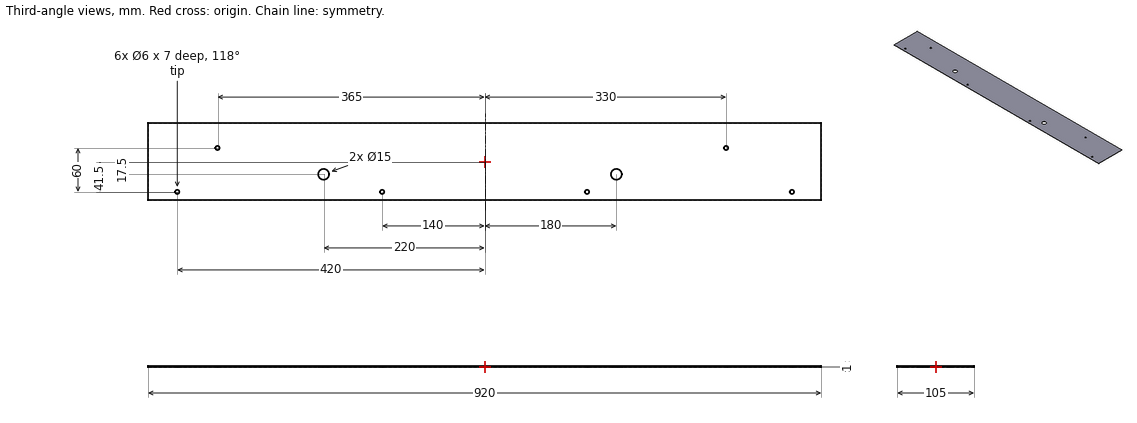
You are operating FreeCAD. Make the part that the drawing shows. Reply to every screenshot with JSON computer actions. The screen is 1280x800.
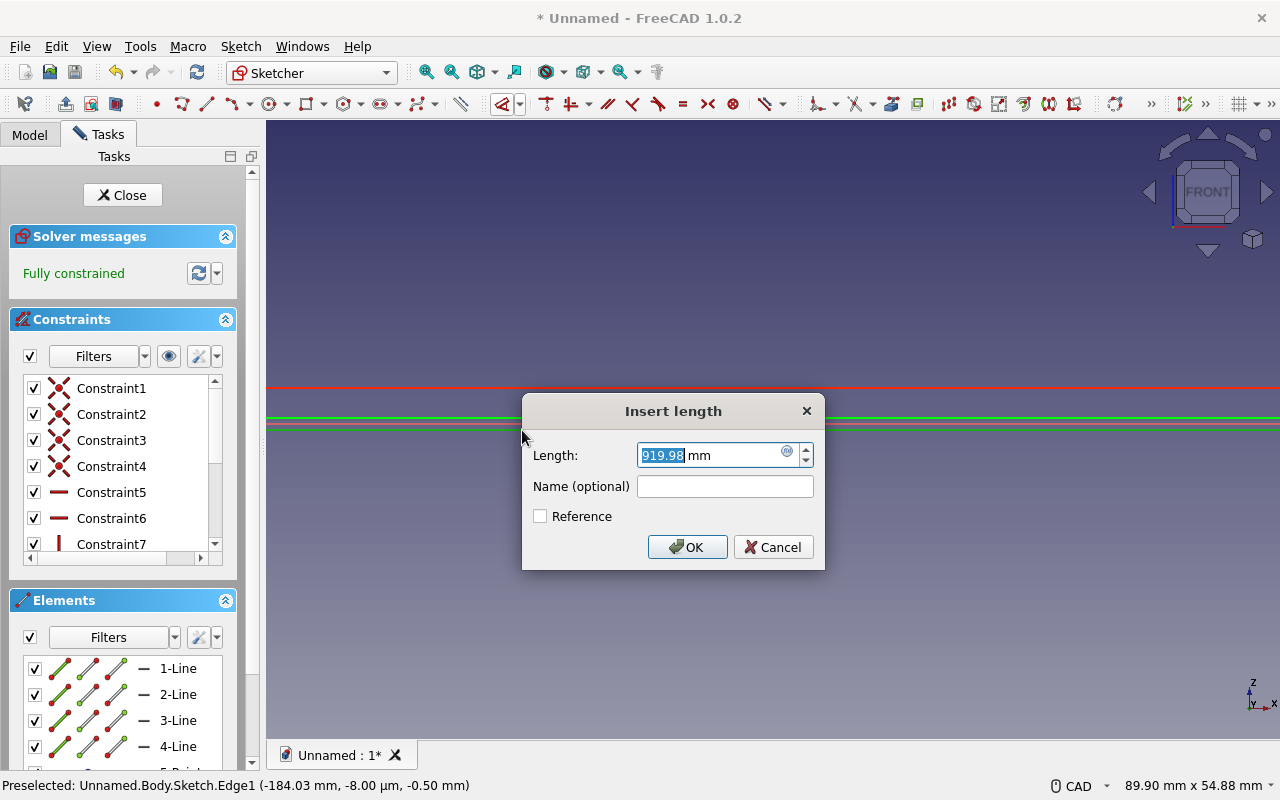
{"action": "type", "text": "920"}
{"action": "key", "text": "Return"}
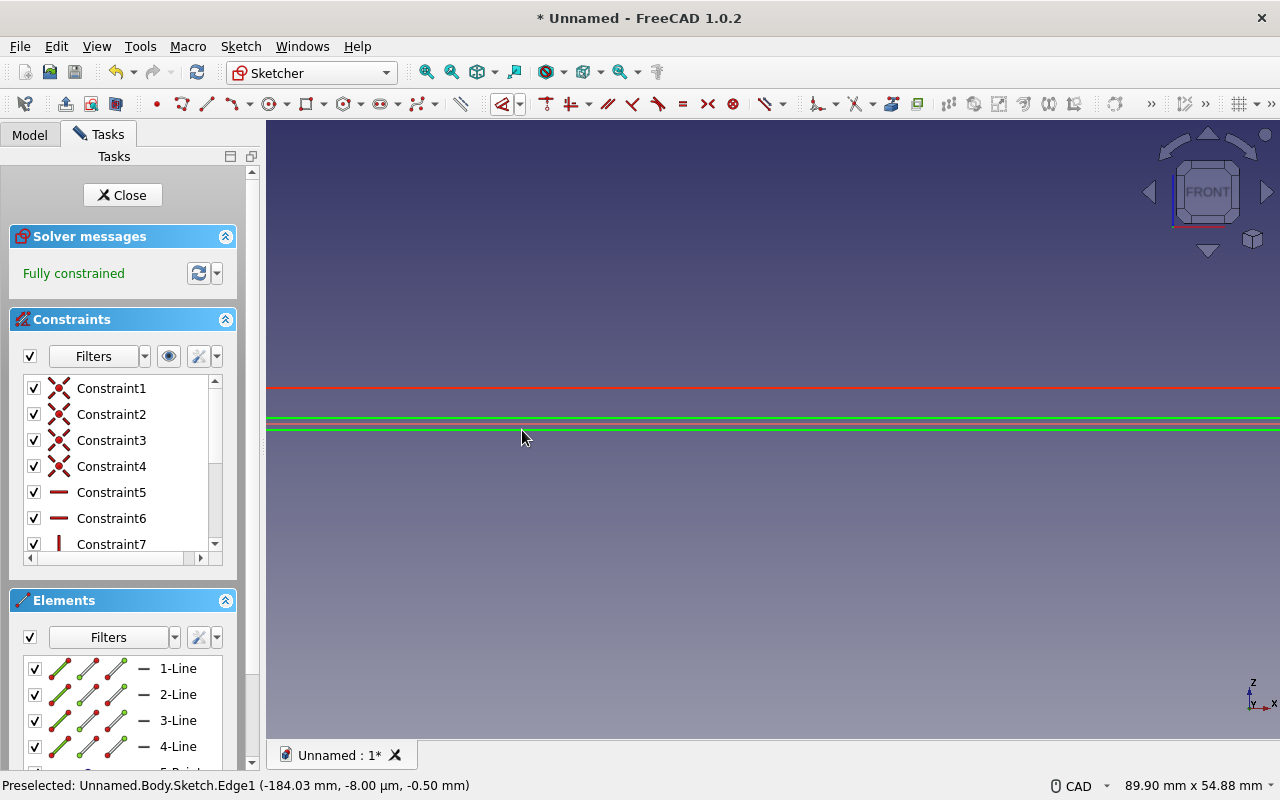
{"action": "left_click", "coordinate": [123, 195]}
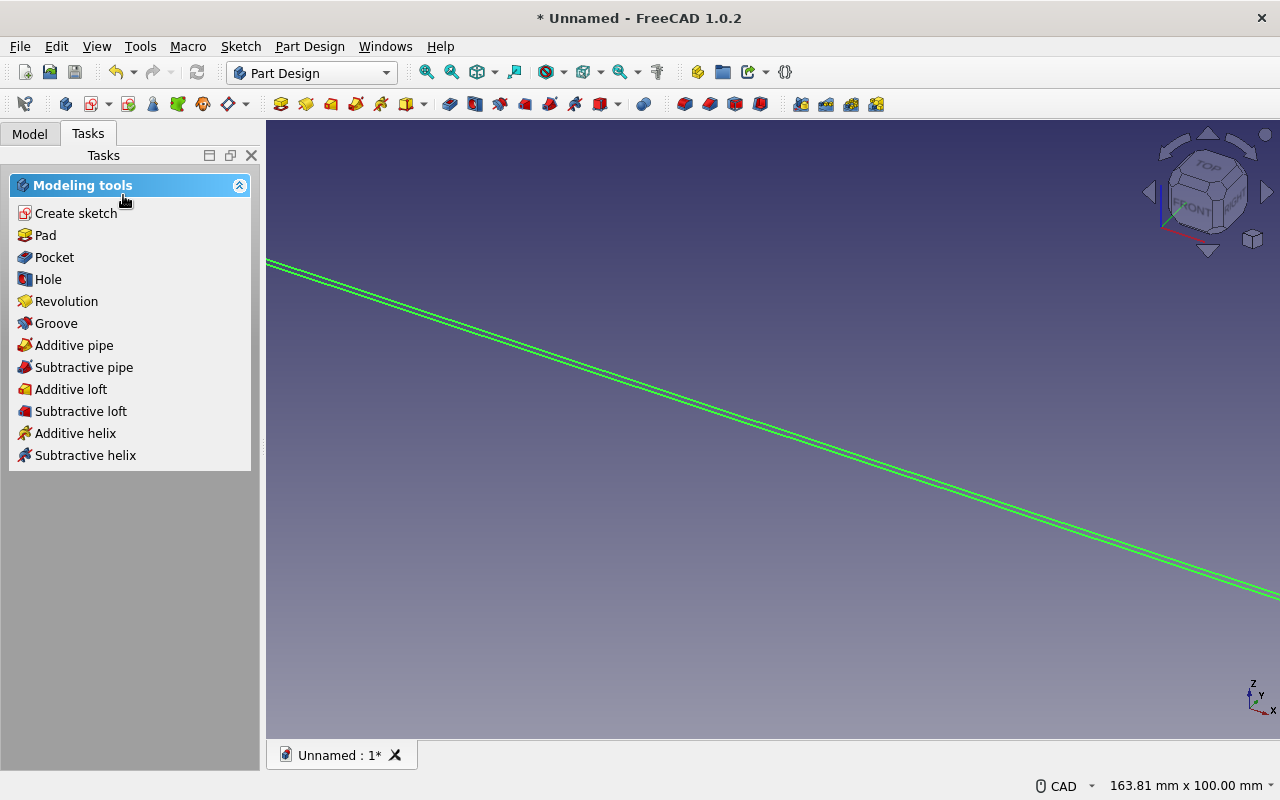
{"action": "left_click", "coordinate": [281, 104]}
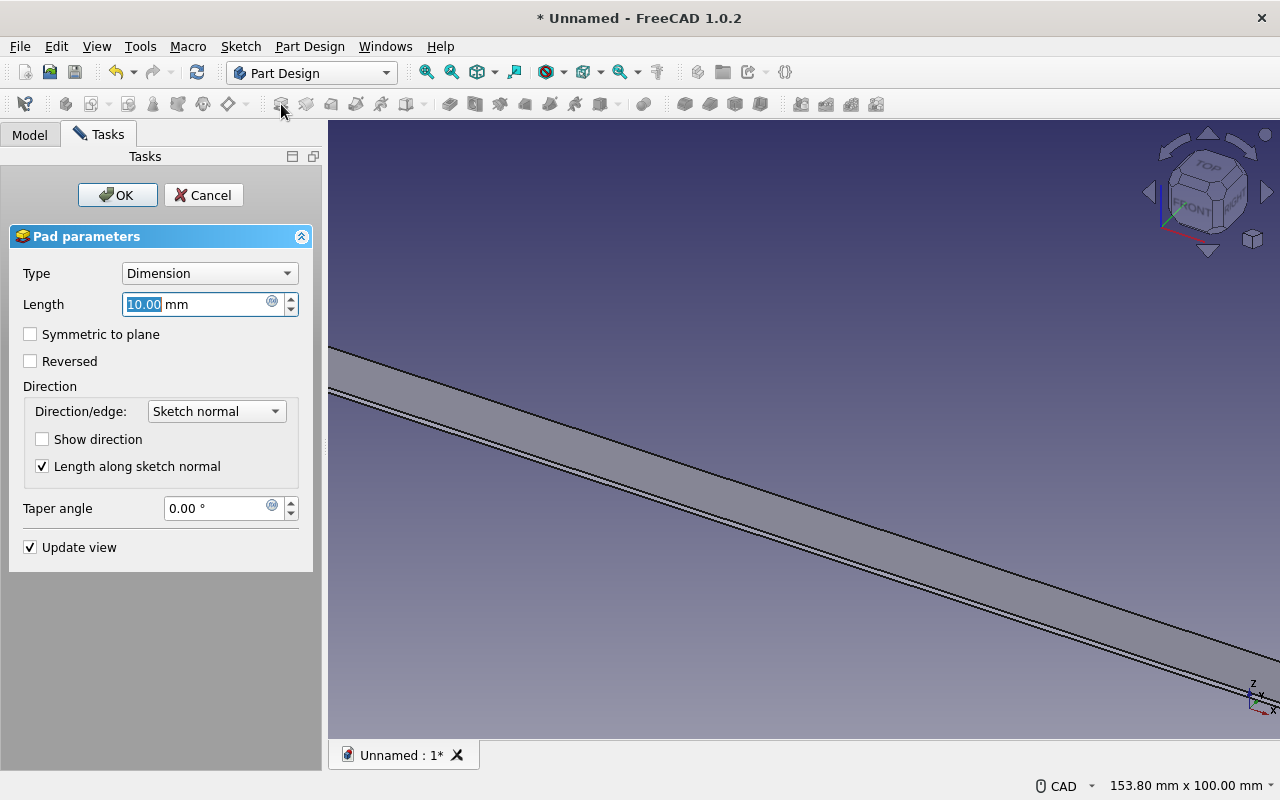
{"action": "type", "text": "105"}
{"action": "key", "text": "Tab"}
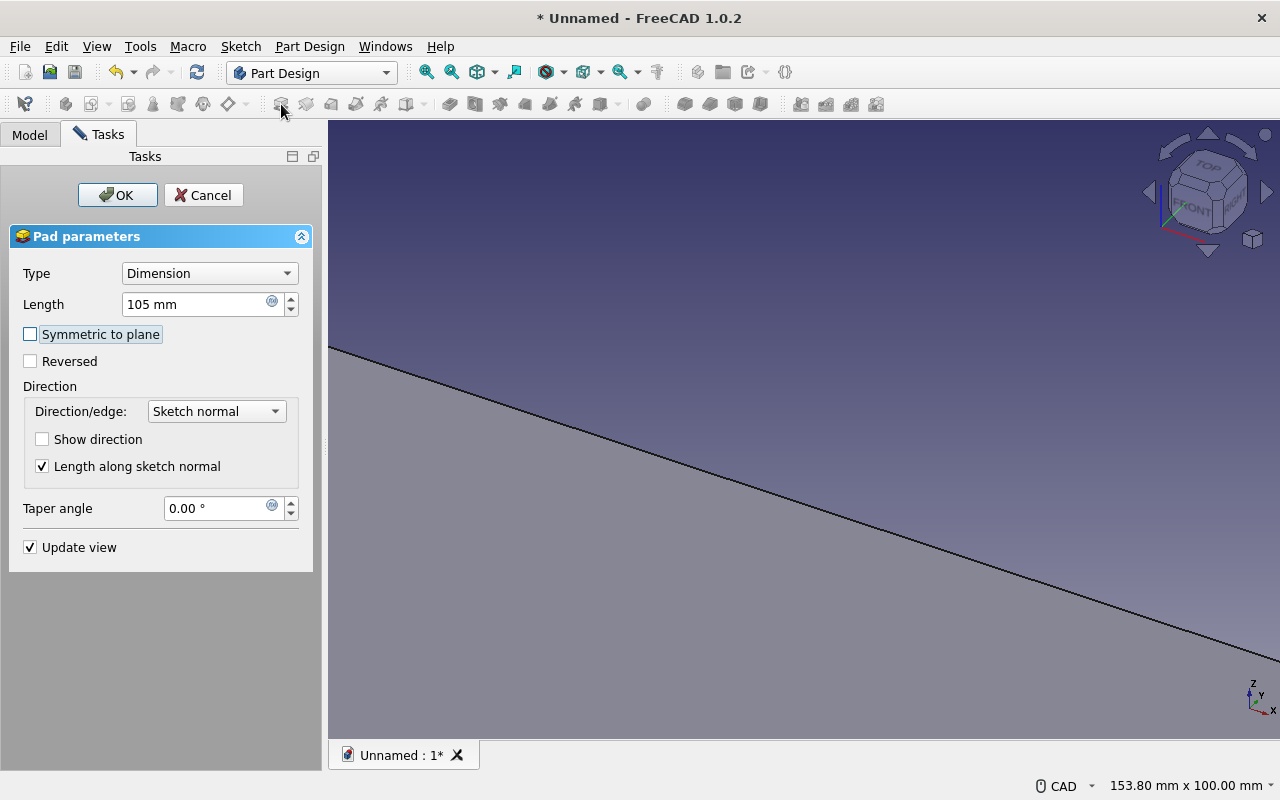
{"action": "left_click", "coordinate": [31, 334]}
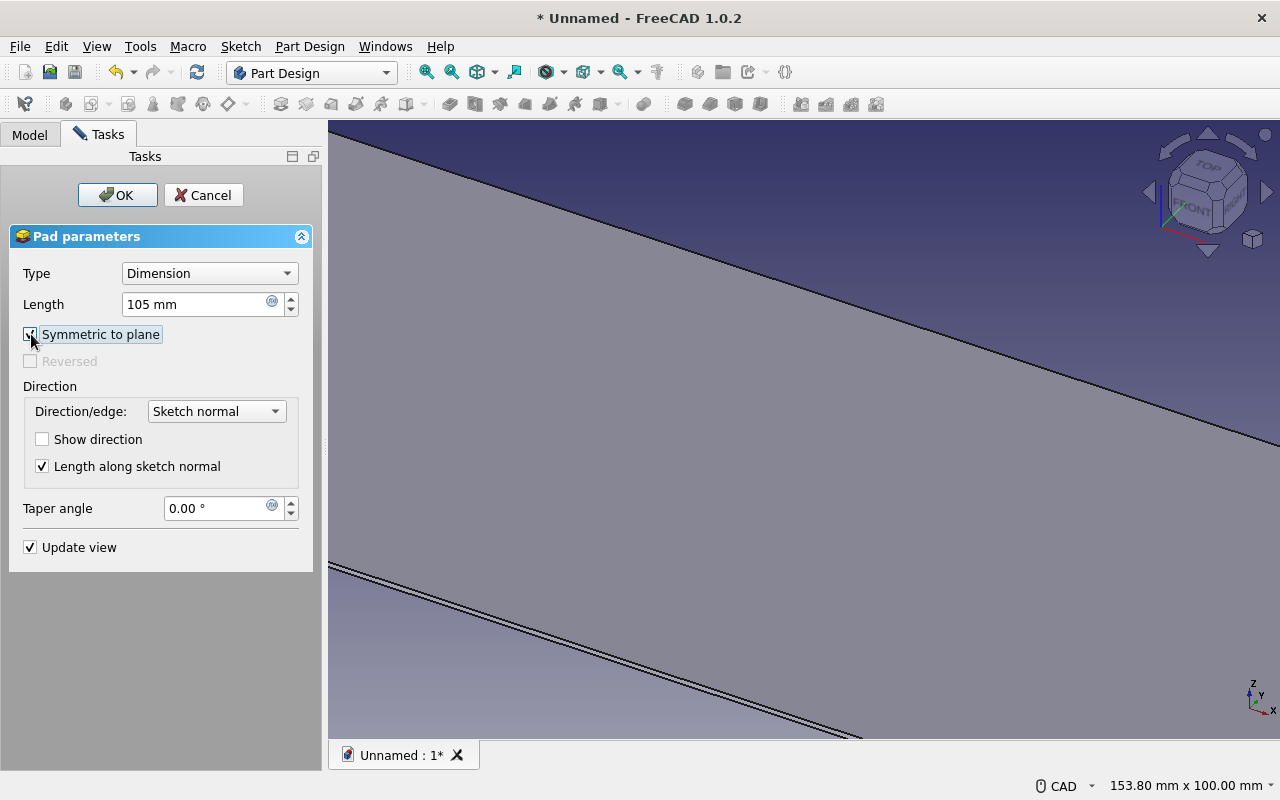
{"action": "left_click", "coordinate": [118, 195]}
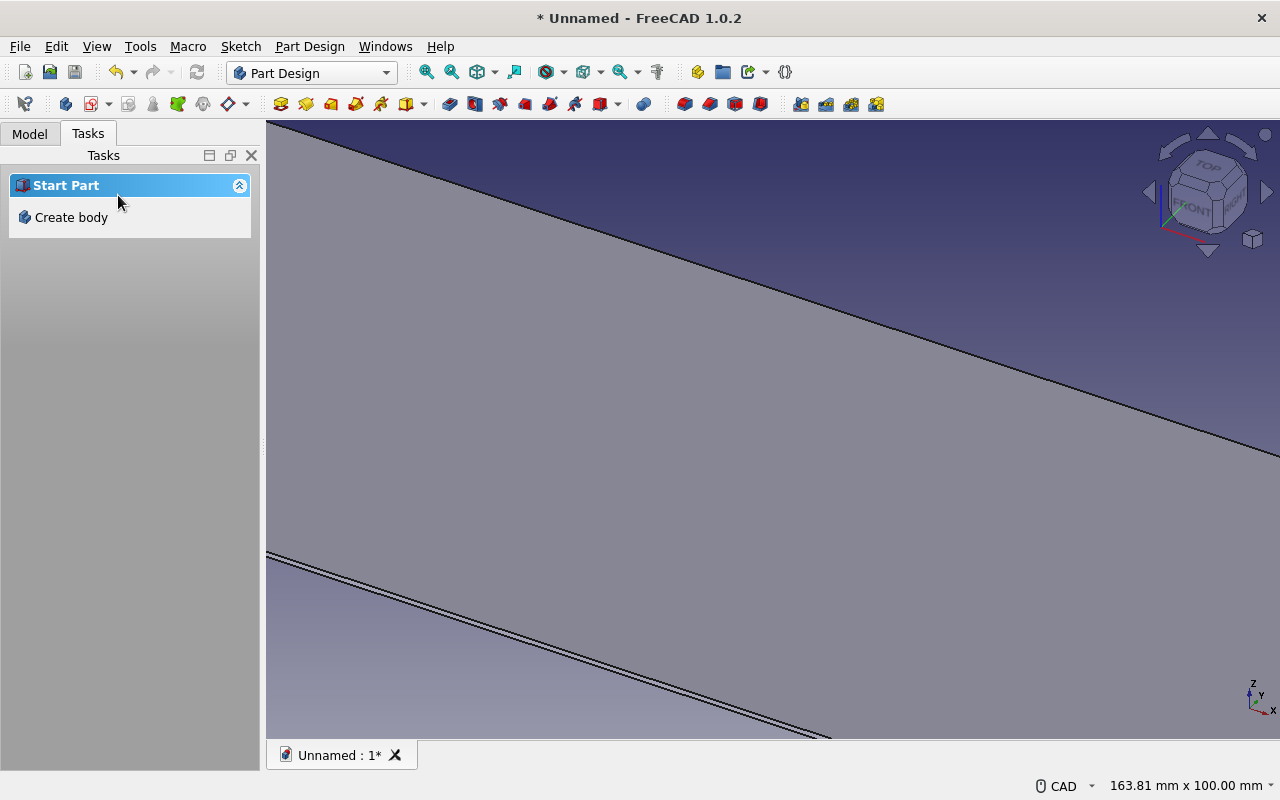
{"action": "left_click", "coordinate": [427, 72]}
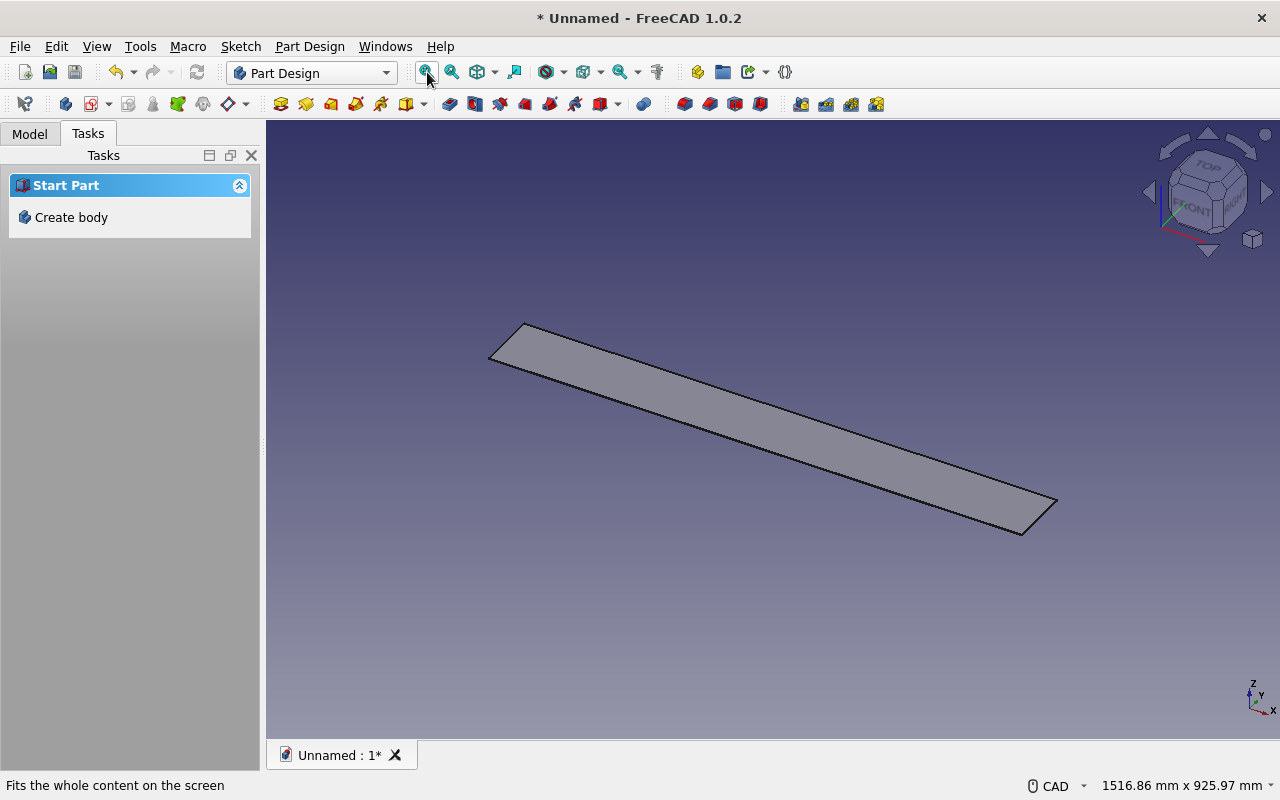
{"action": "left_click", "coordinate": [1001, 504]}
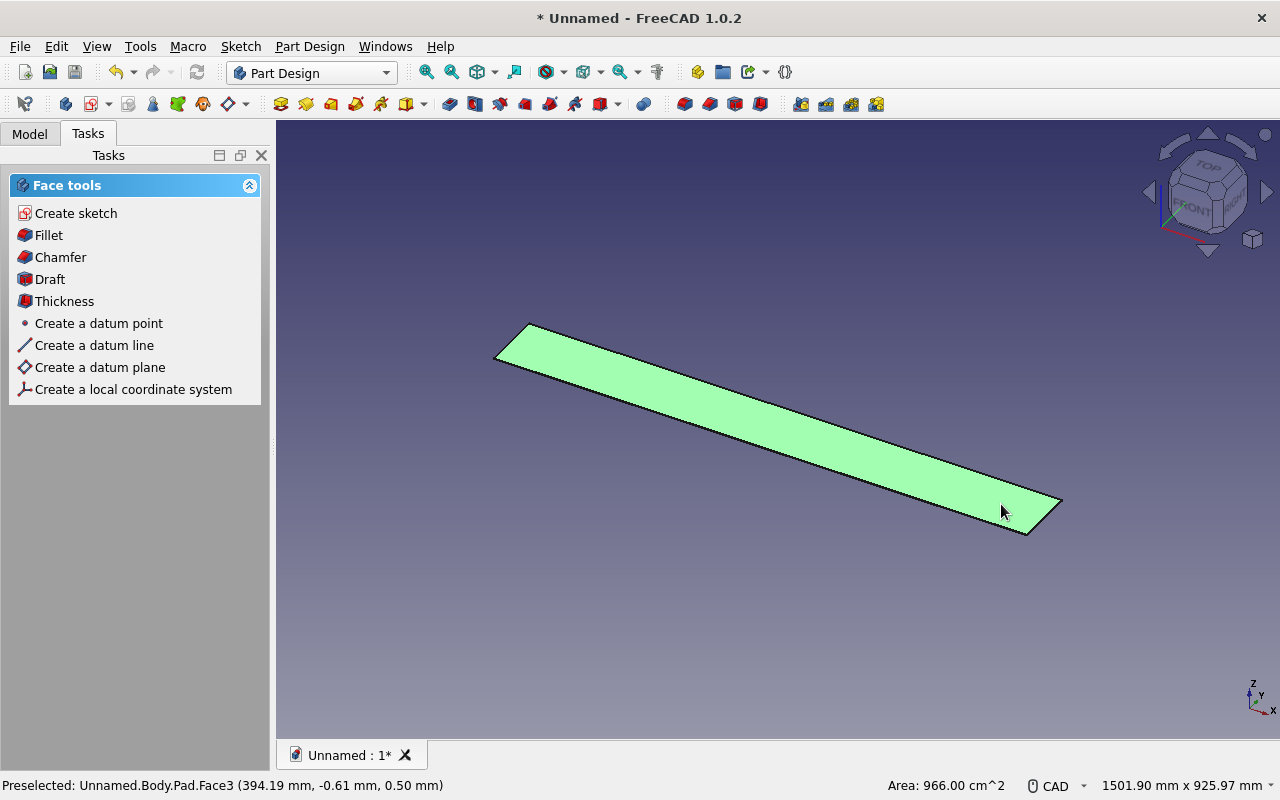
{"action": "left_click", "coordinate": [90, 104]}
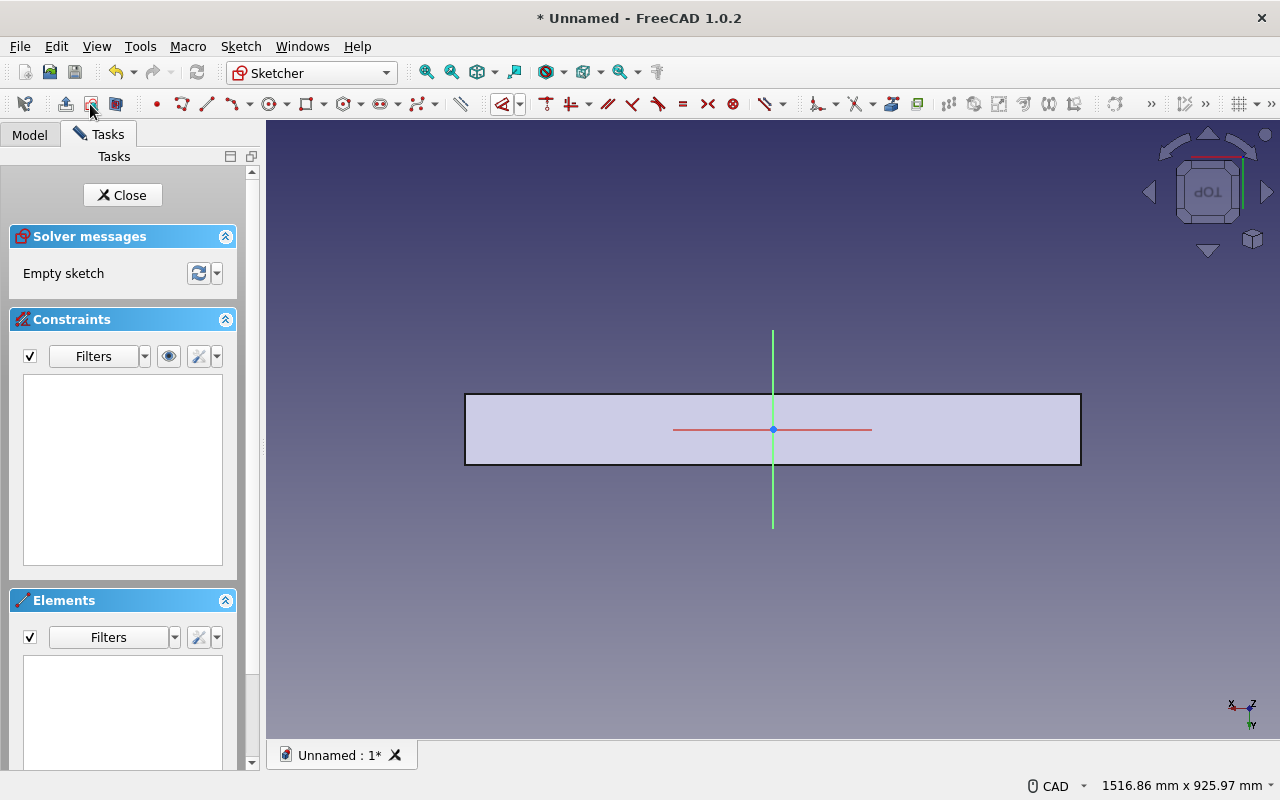
{"action": "scroll", "coordinate": [853, 414], "scroll_direction": "up", "scroll_amount": 4}